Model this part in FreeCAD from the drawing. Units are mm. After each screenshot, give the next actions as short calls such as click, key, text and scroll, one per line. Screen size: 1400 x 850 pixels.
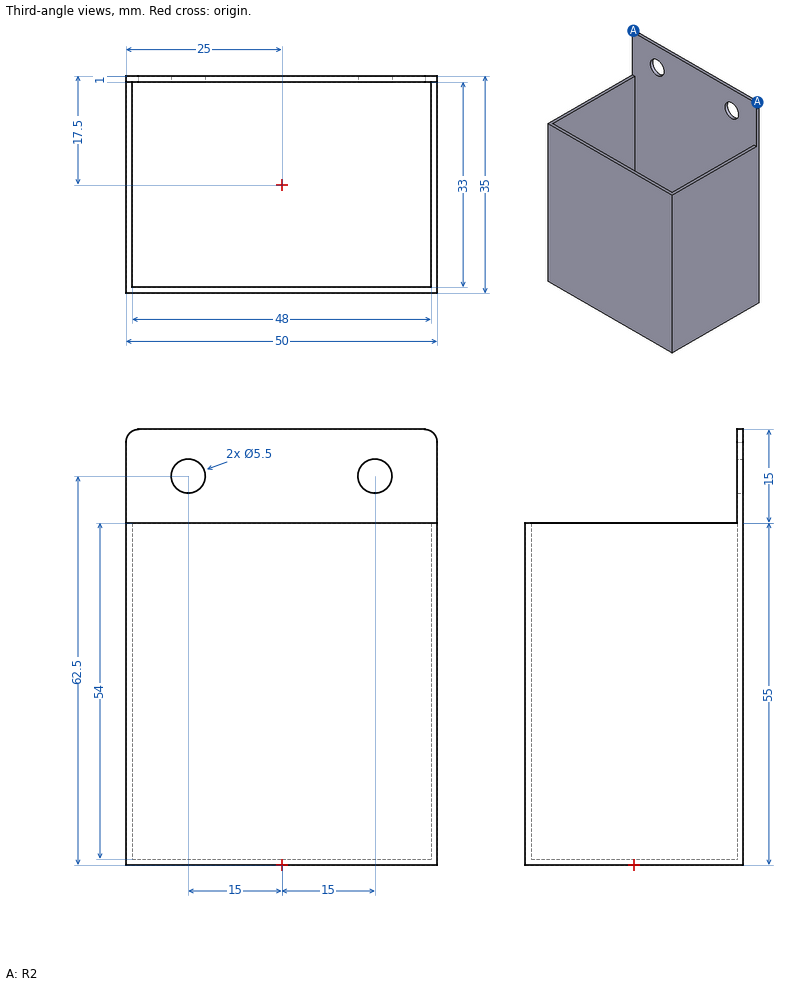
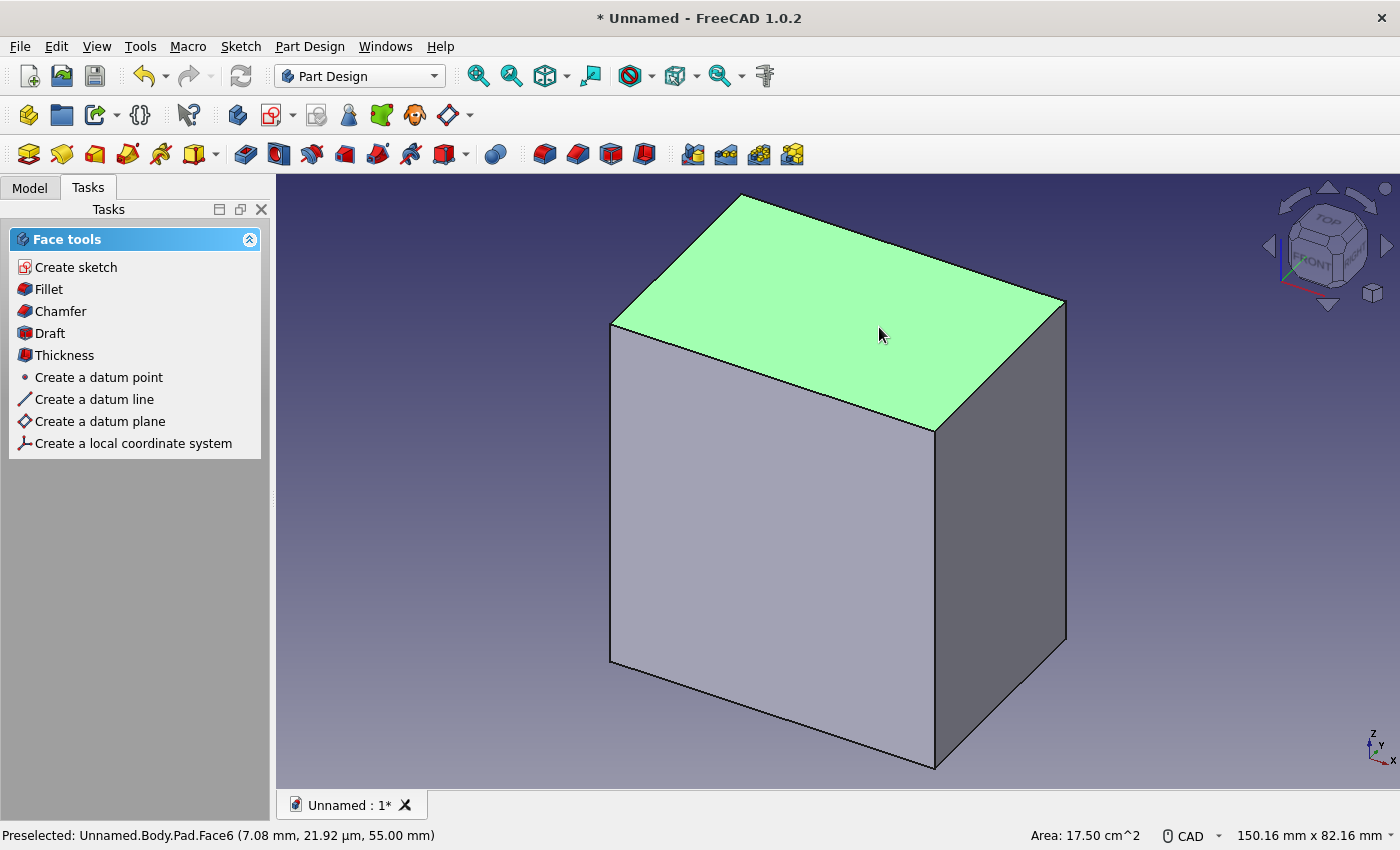
click(270, 116)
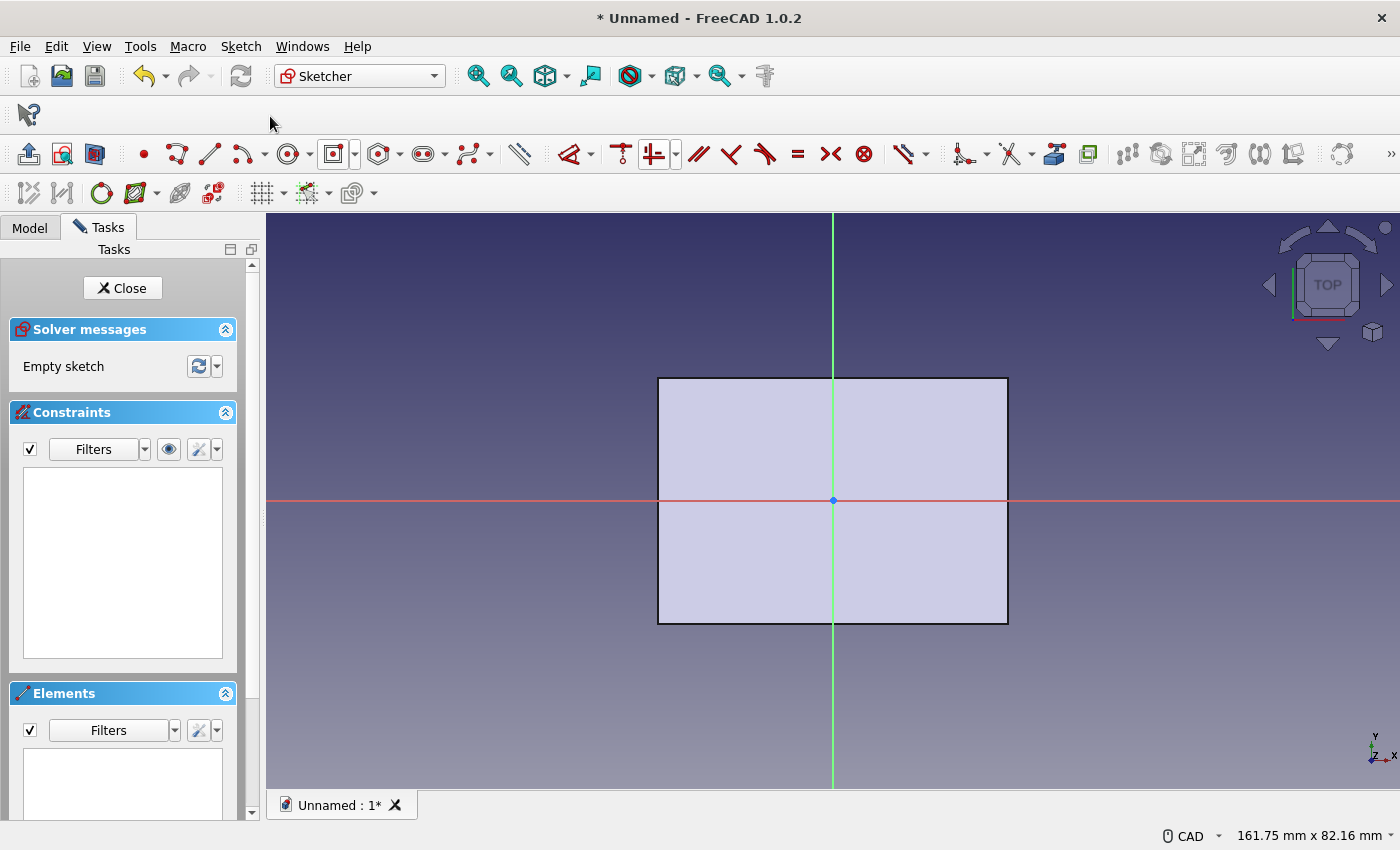
scroll(972, 501, up, 2)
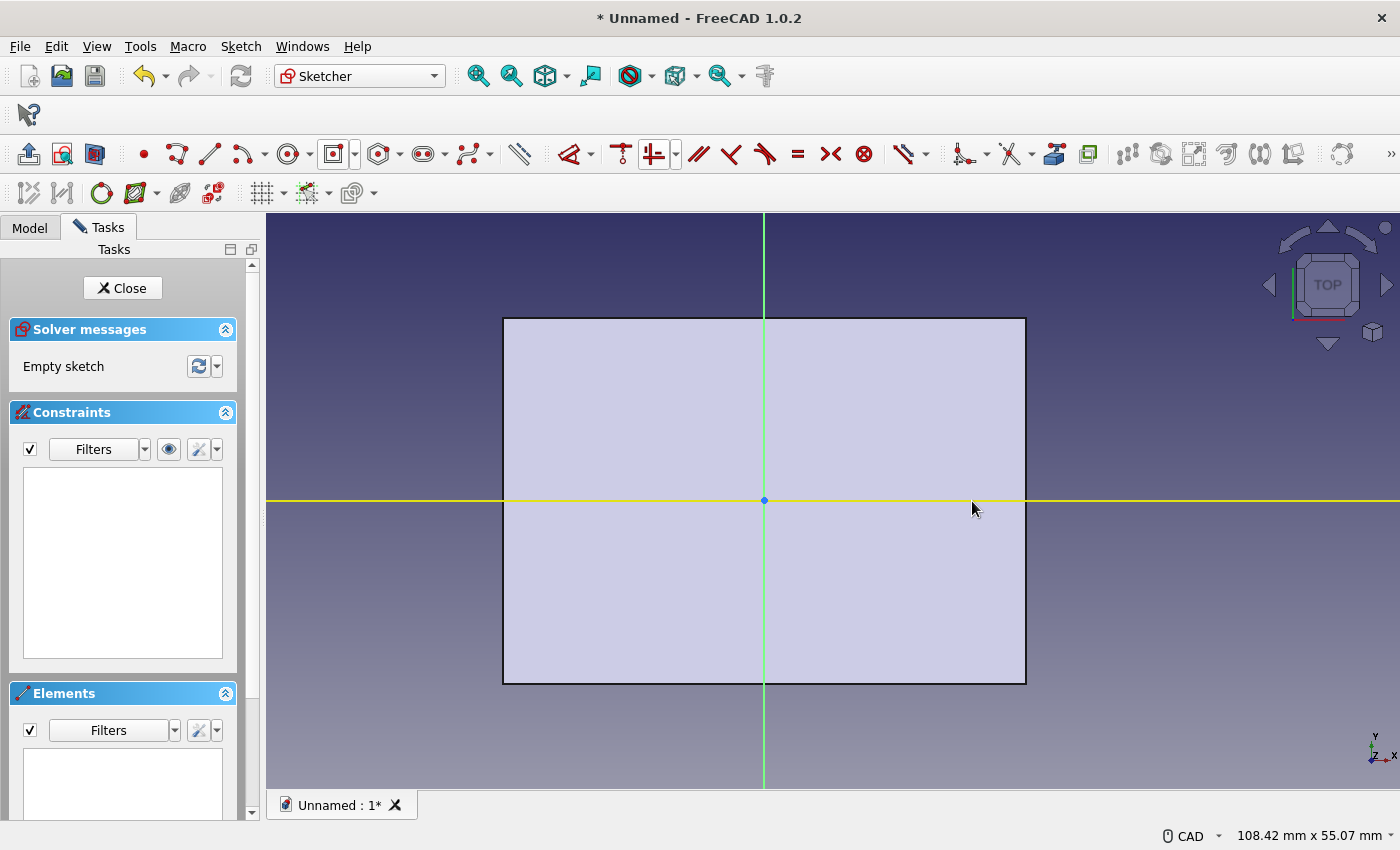
click(332, 154)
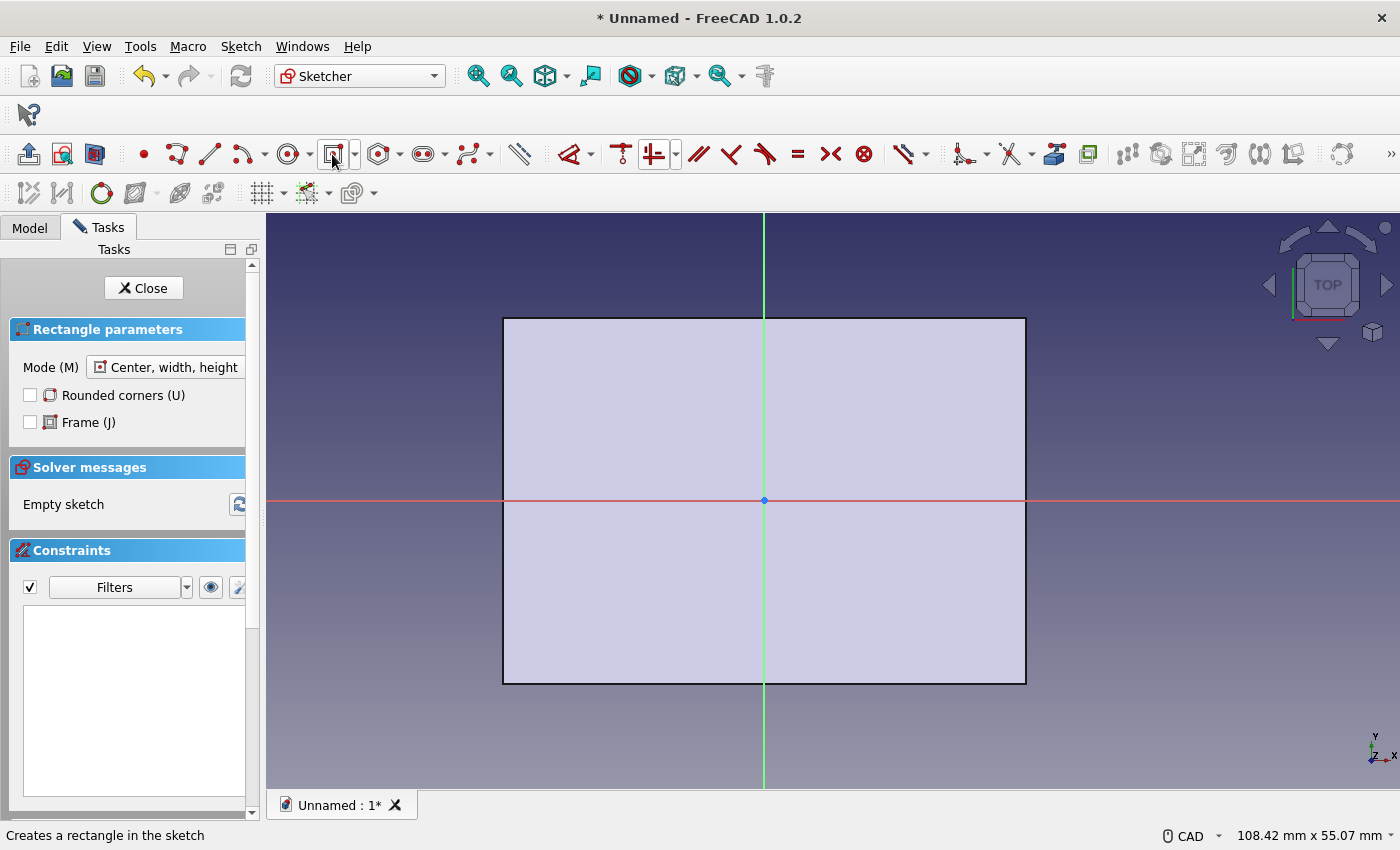
click(764, 501)
click(1015, 328)
key(Escape)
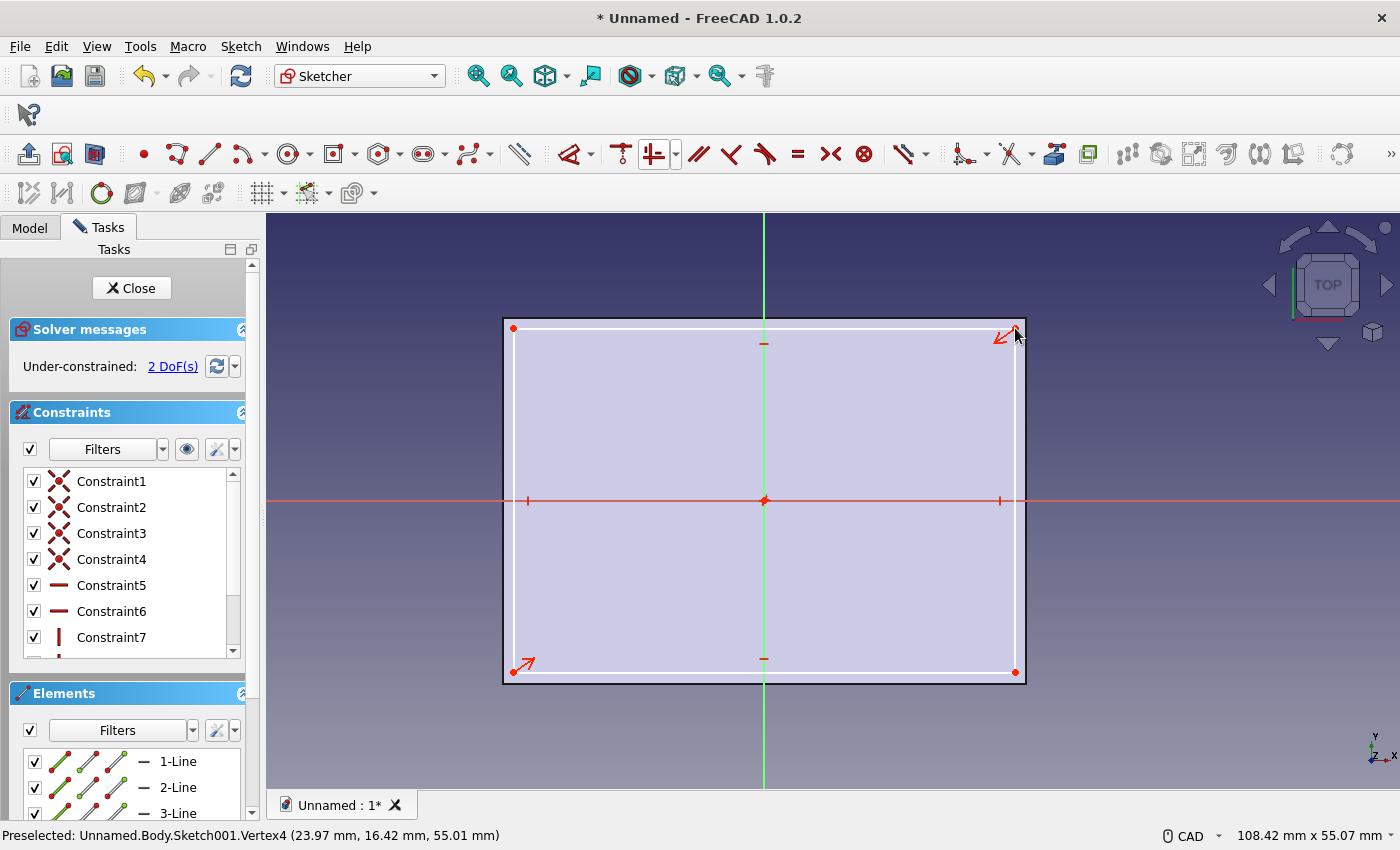
click(568, 154)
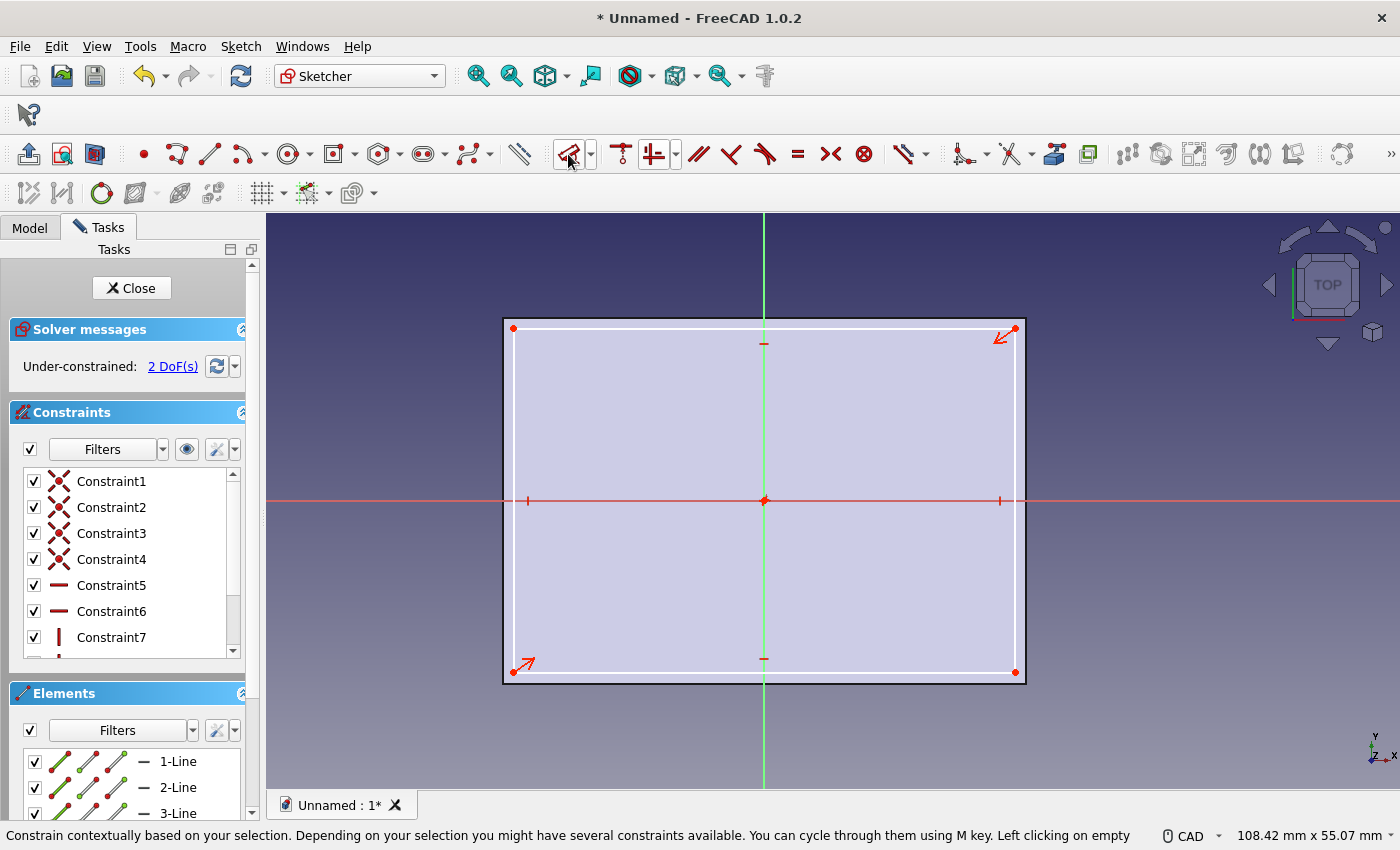
click(664, 673)
click(649, 707)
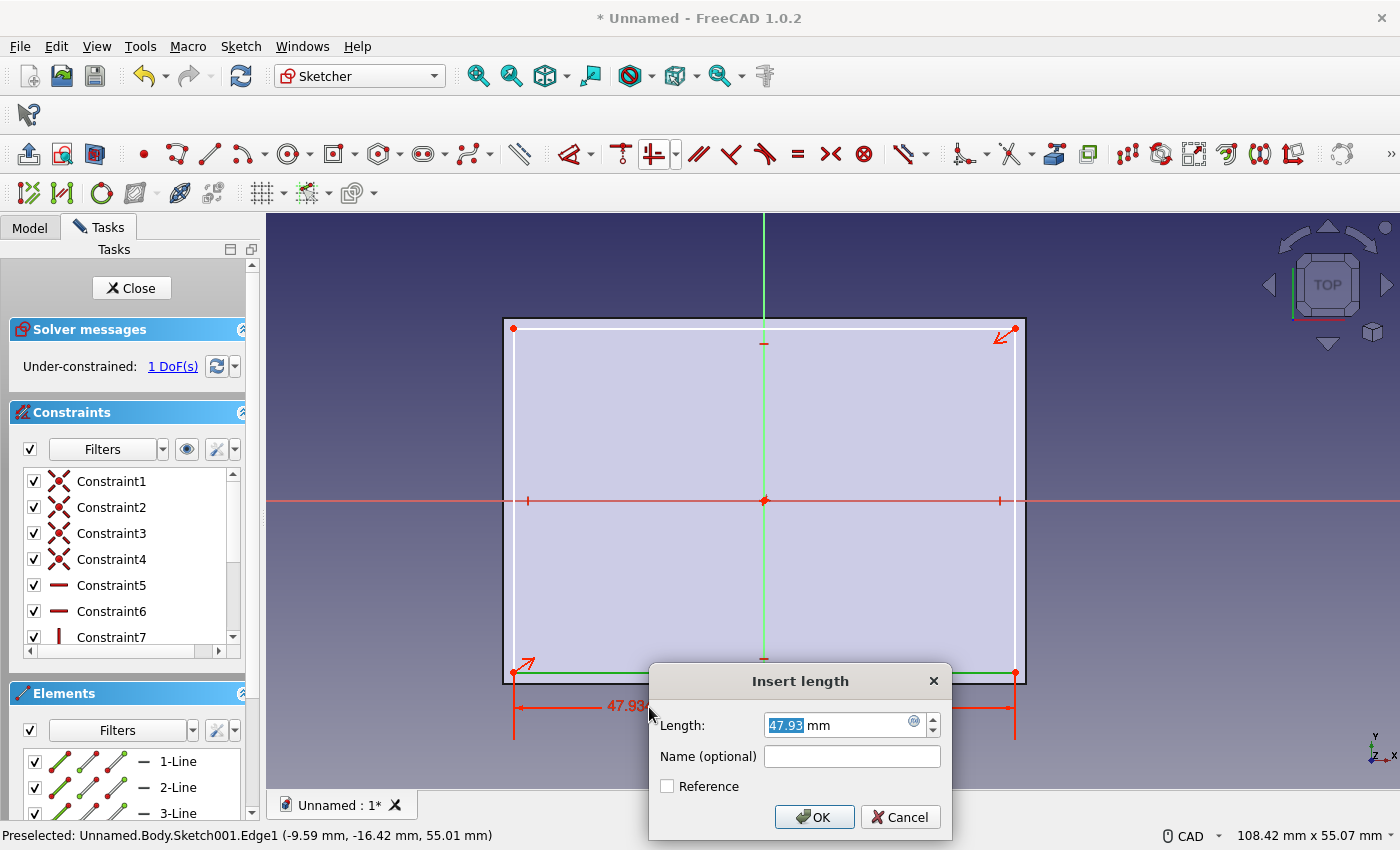
text(48)
key(Return)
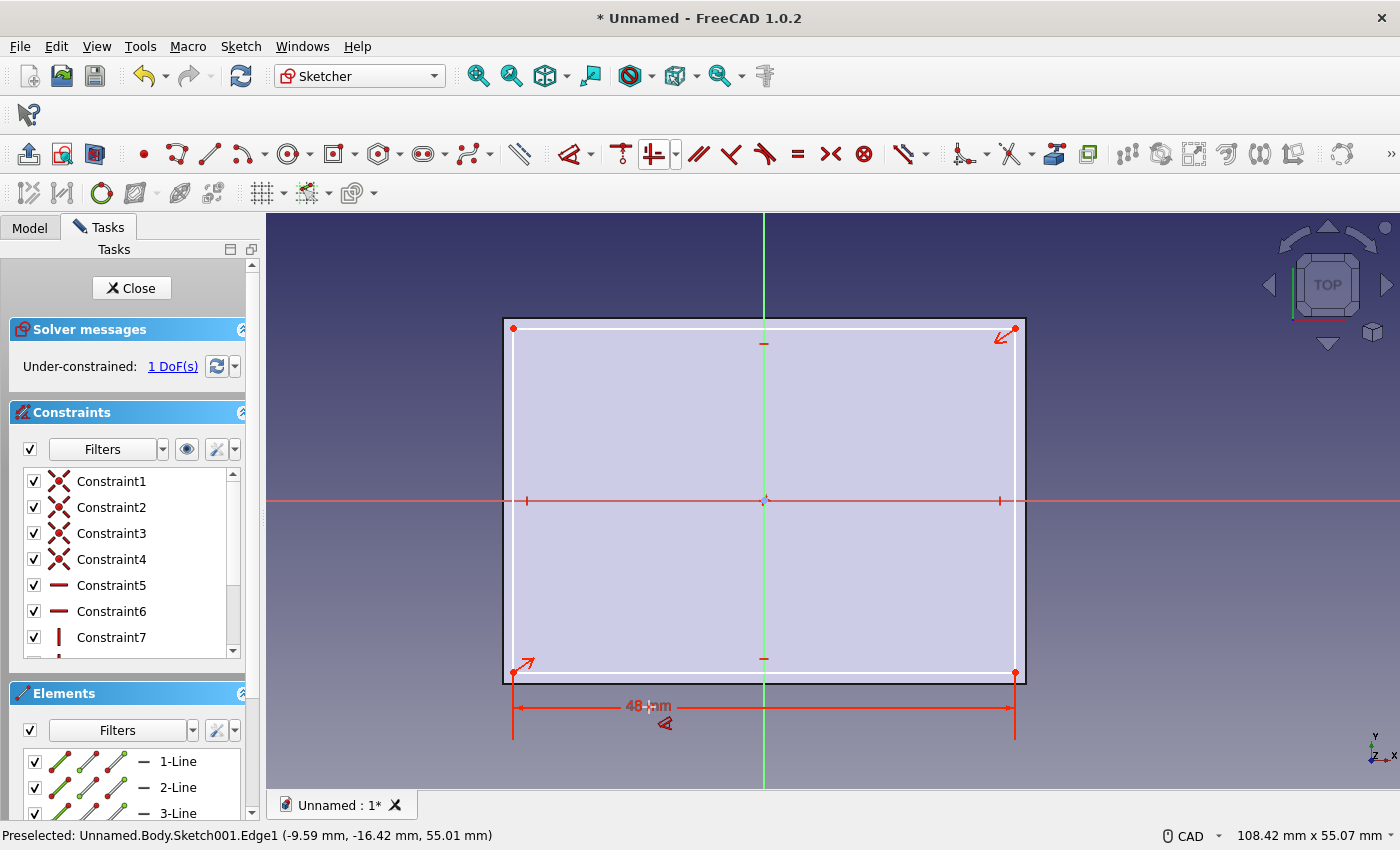
click(1015, 569)
click(1049, 422)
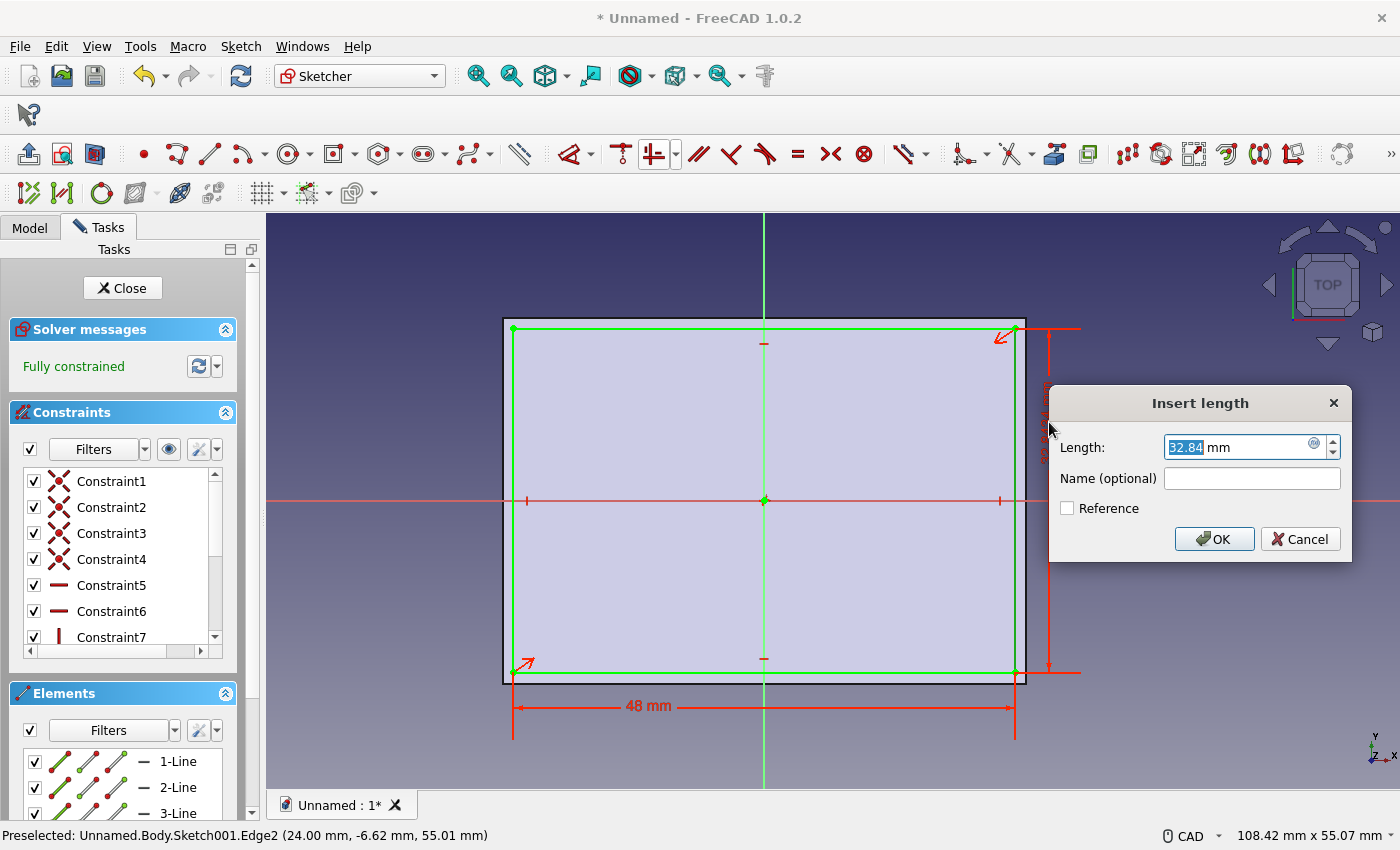
text(33)
key(Return)
key(Escape)